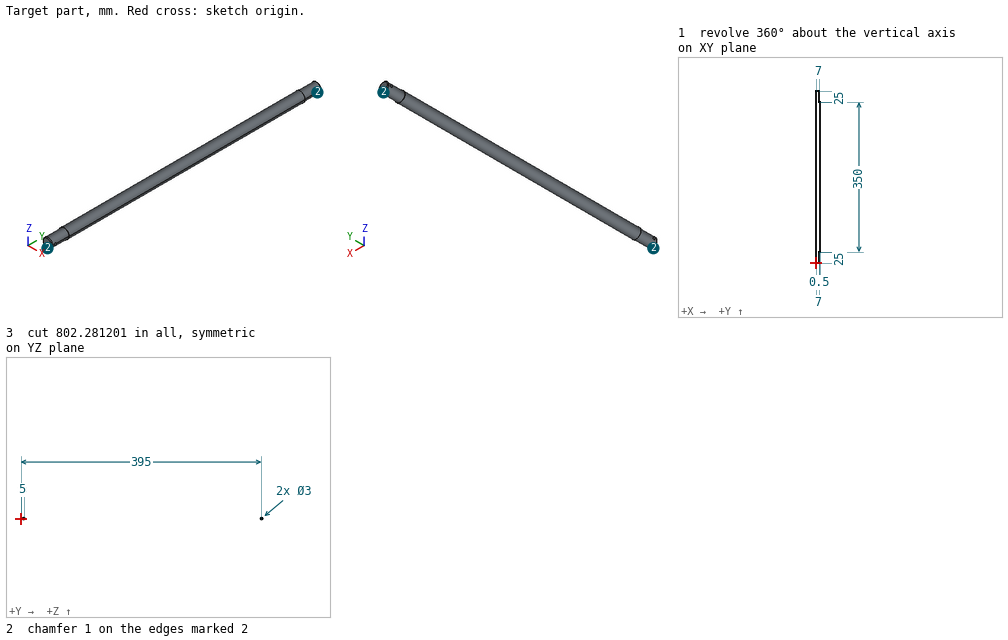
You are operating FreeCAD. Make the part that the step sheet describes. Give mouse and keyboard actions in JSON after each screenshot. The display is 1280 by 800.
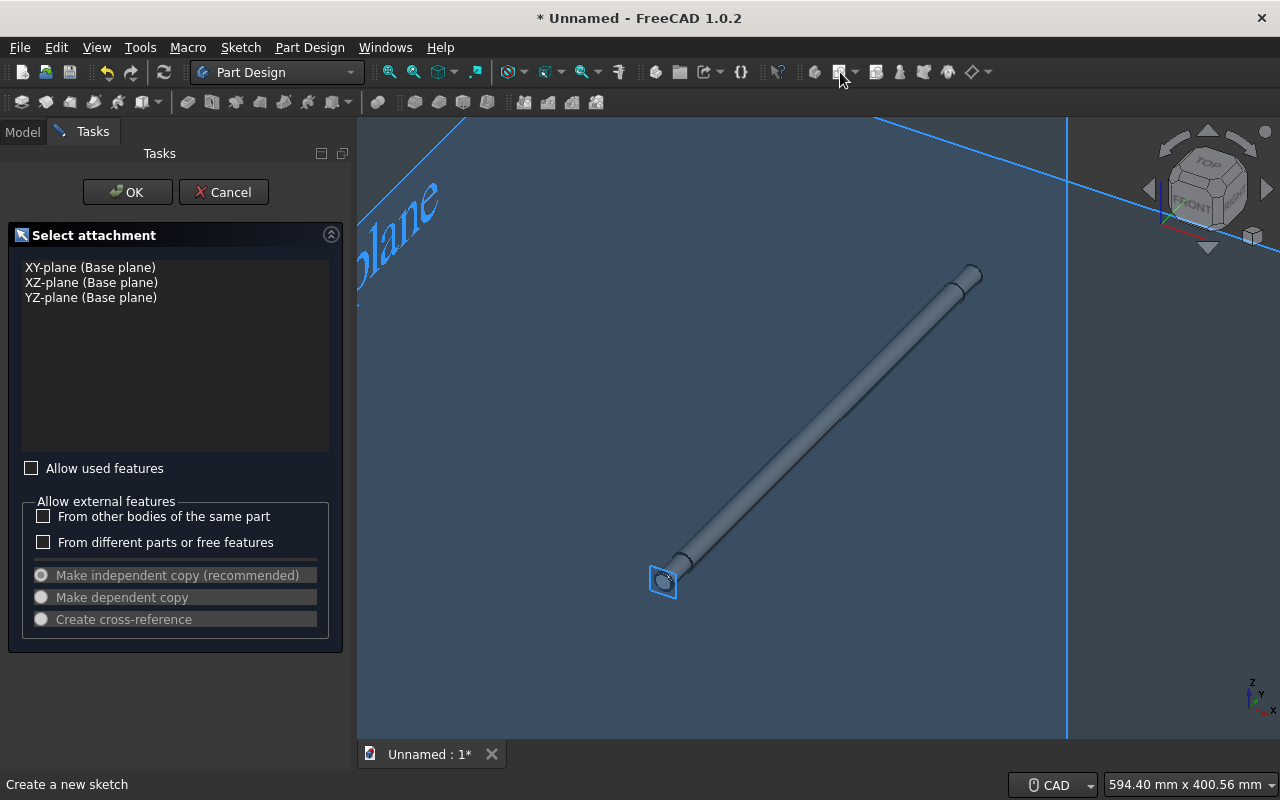
{"action": "left_click", "coordinate": [82, 298]}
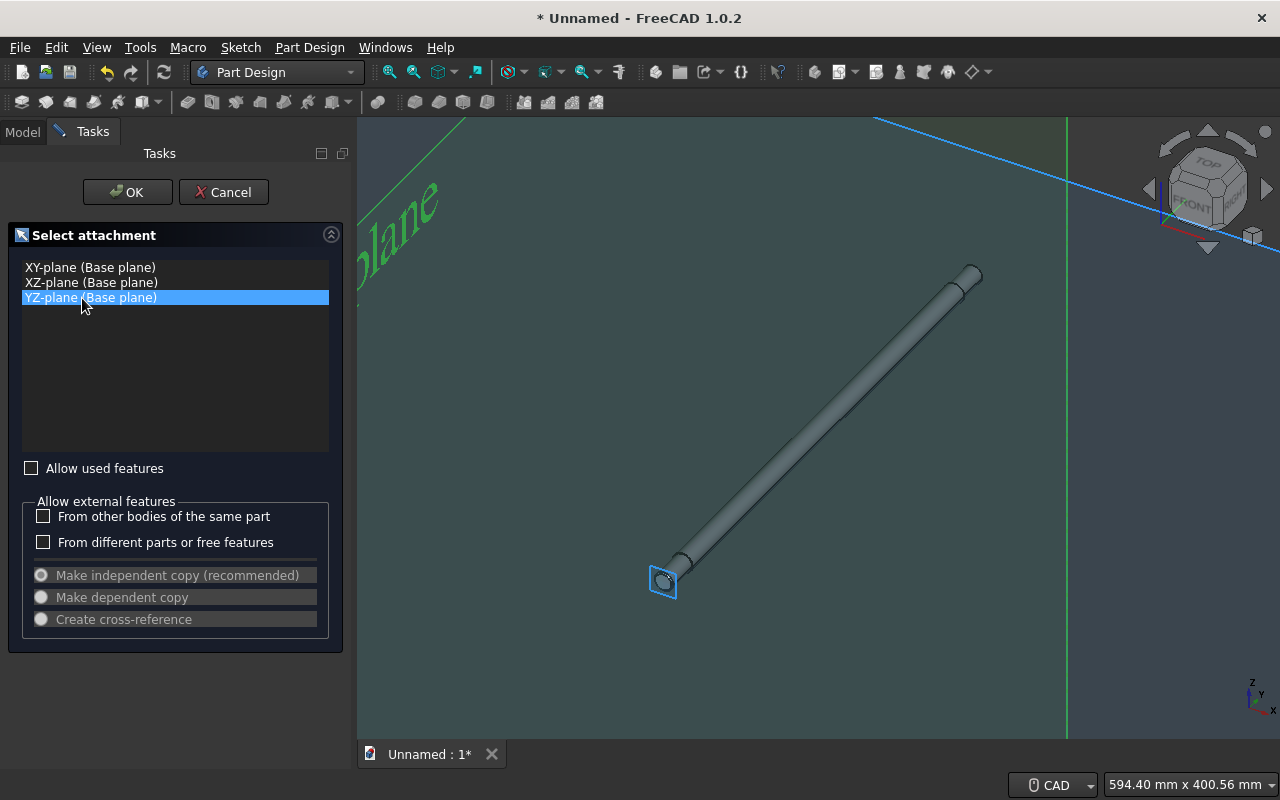
{"action": "left_click", "coordinate": [128, 192]}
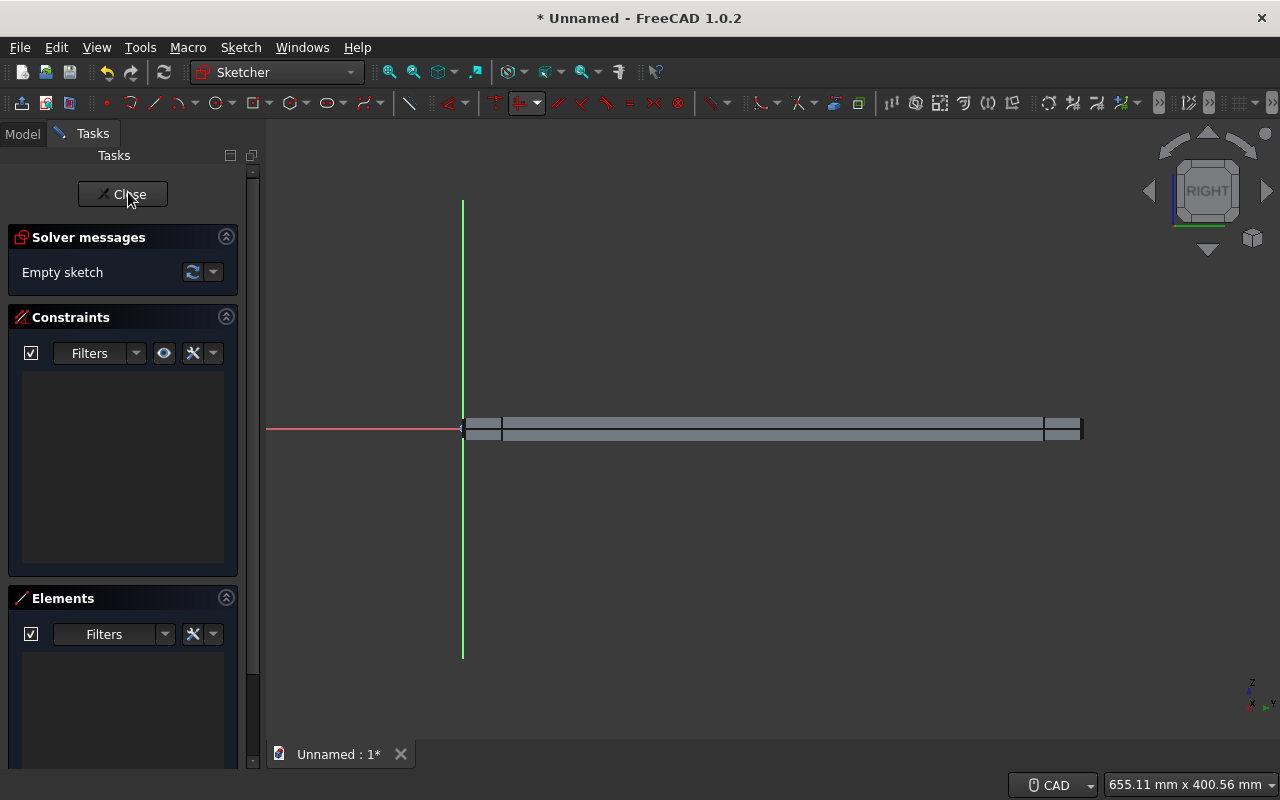
{"action": "left_click", "coordinate": [70, 104]}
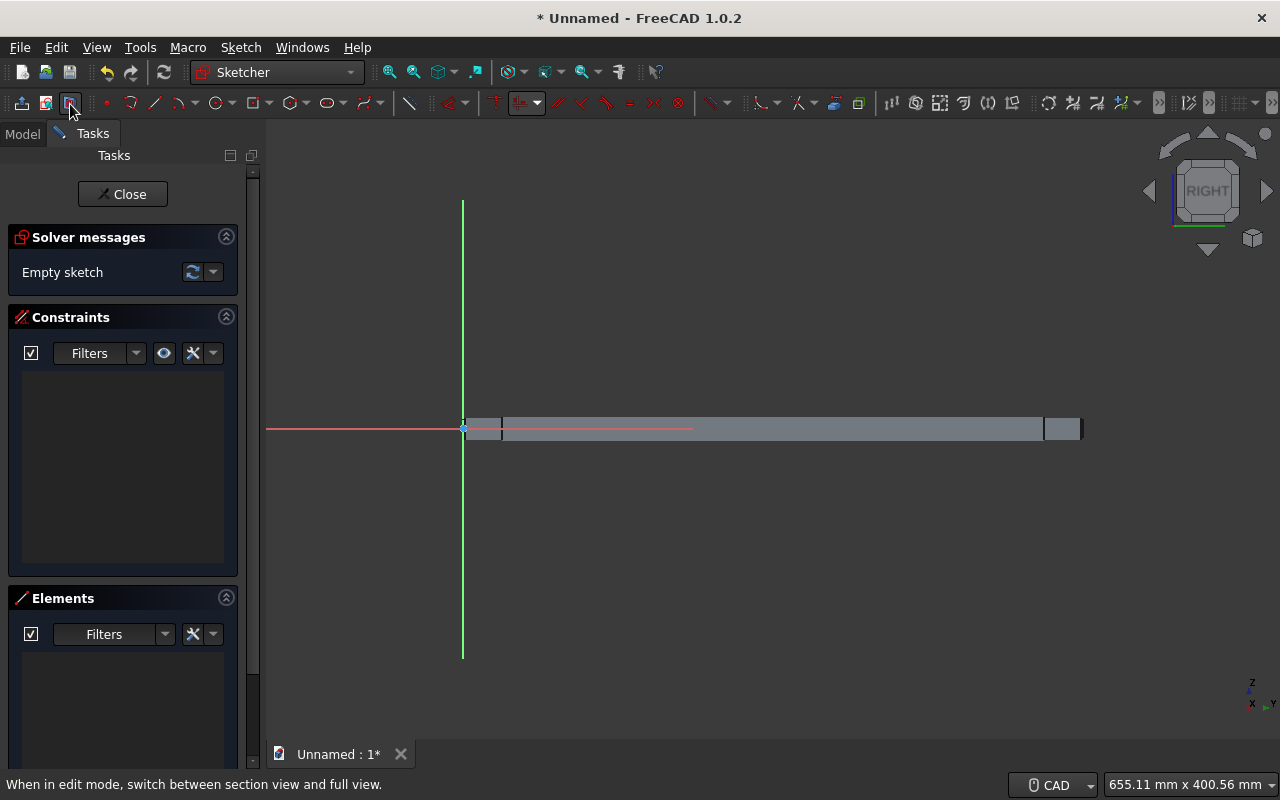
{"action": "key", "text": "g c"}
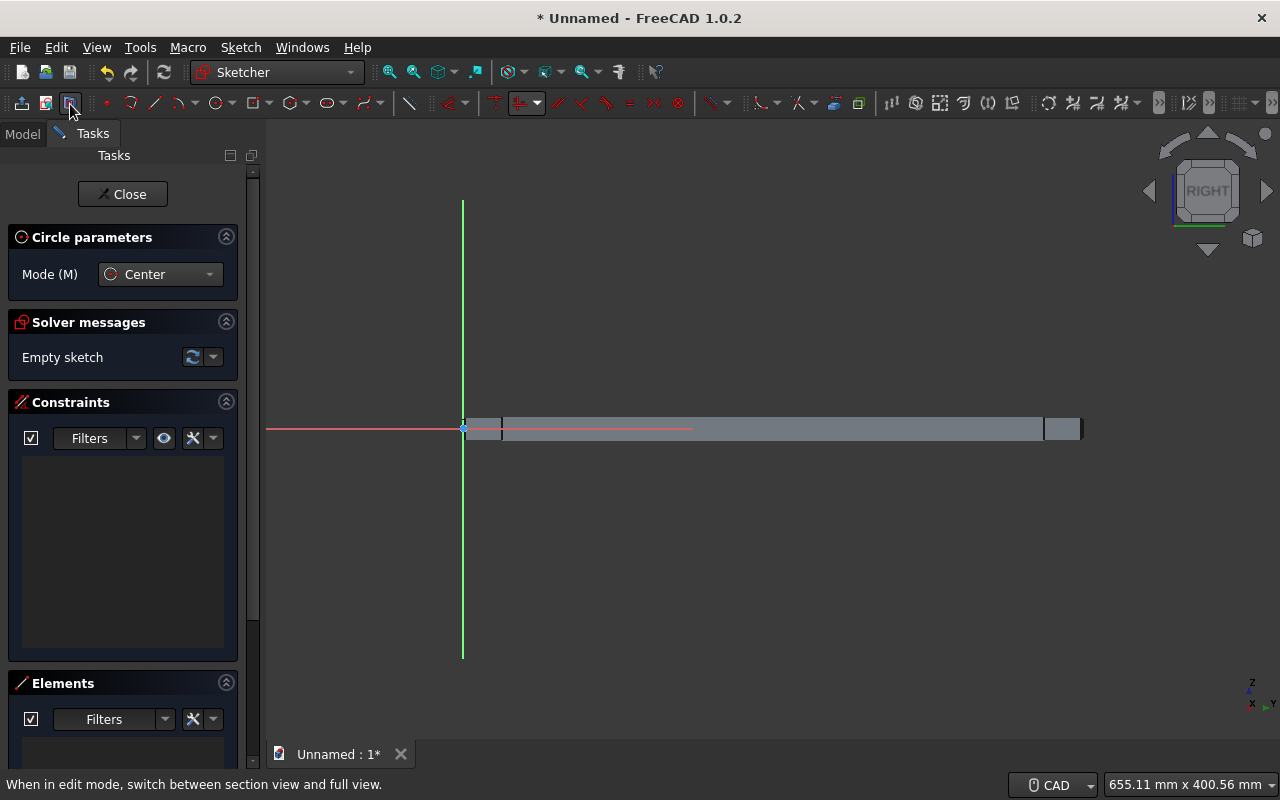
{"action": "scroll", "coordinate": [1075, 429], "scroll_direction": "up", "scroll_amount": 12}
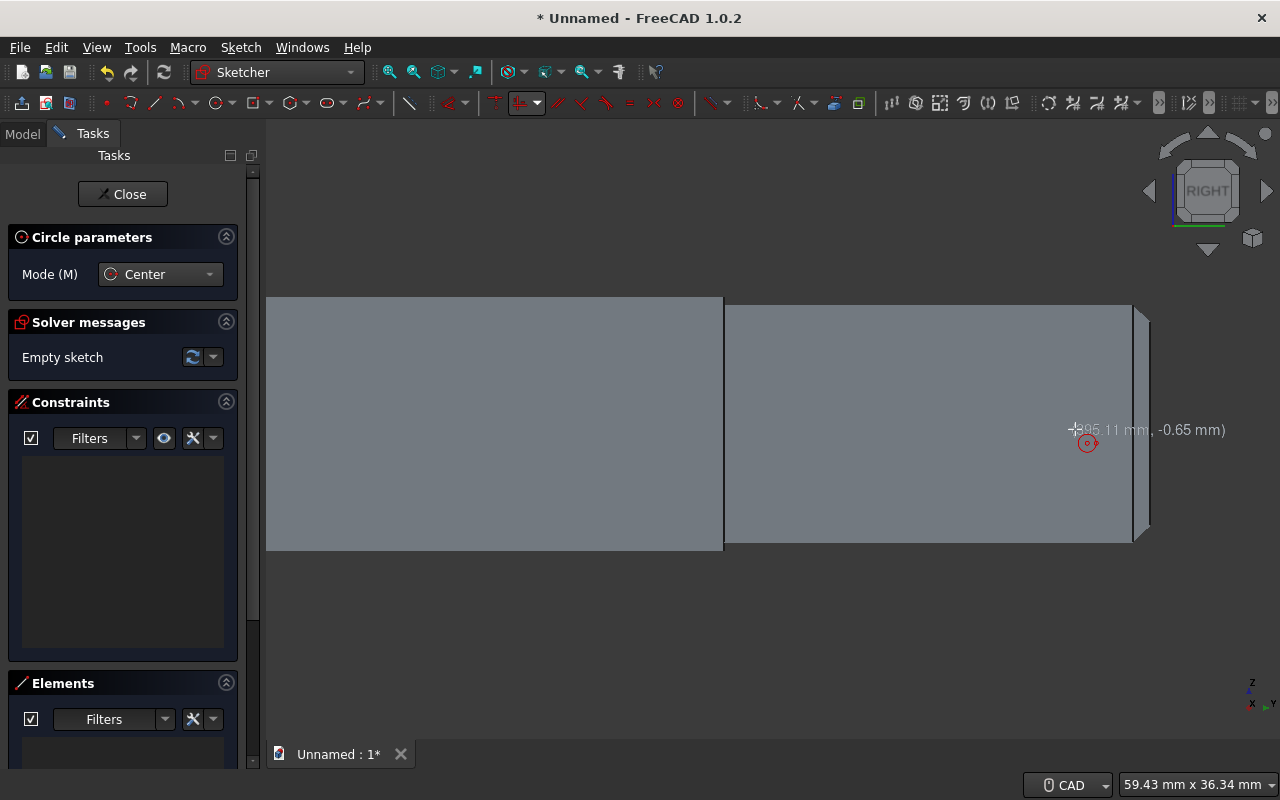
{"action": "scroll", "coordinate": [1003, 430], "scroll_direction": "down", "scroll_amount": 12}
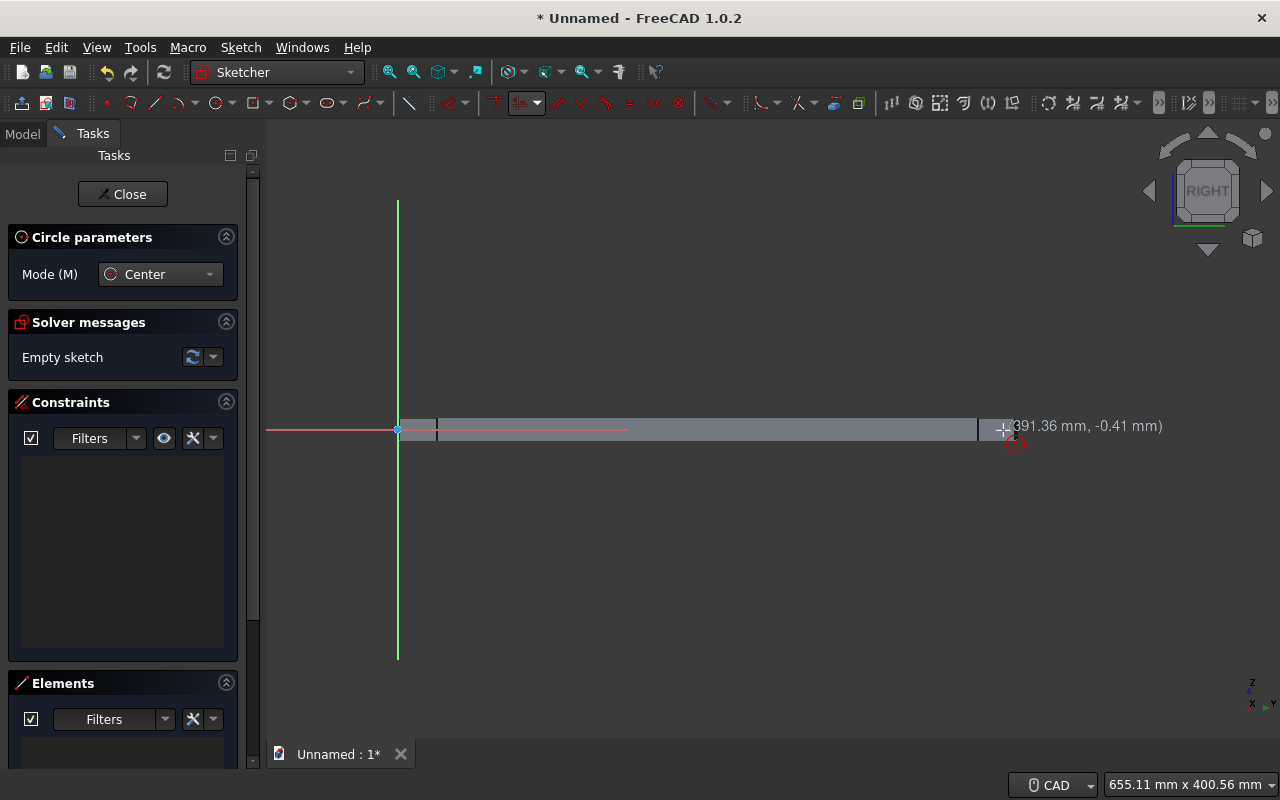
{"action": "left_click", "coordinate": [1009, 430]}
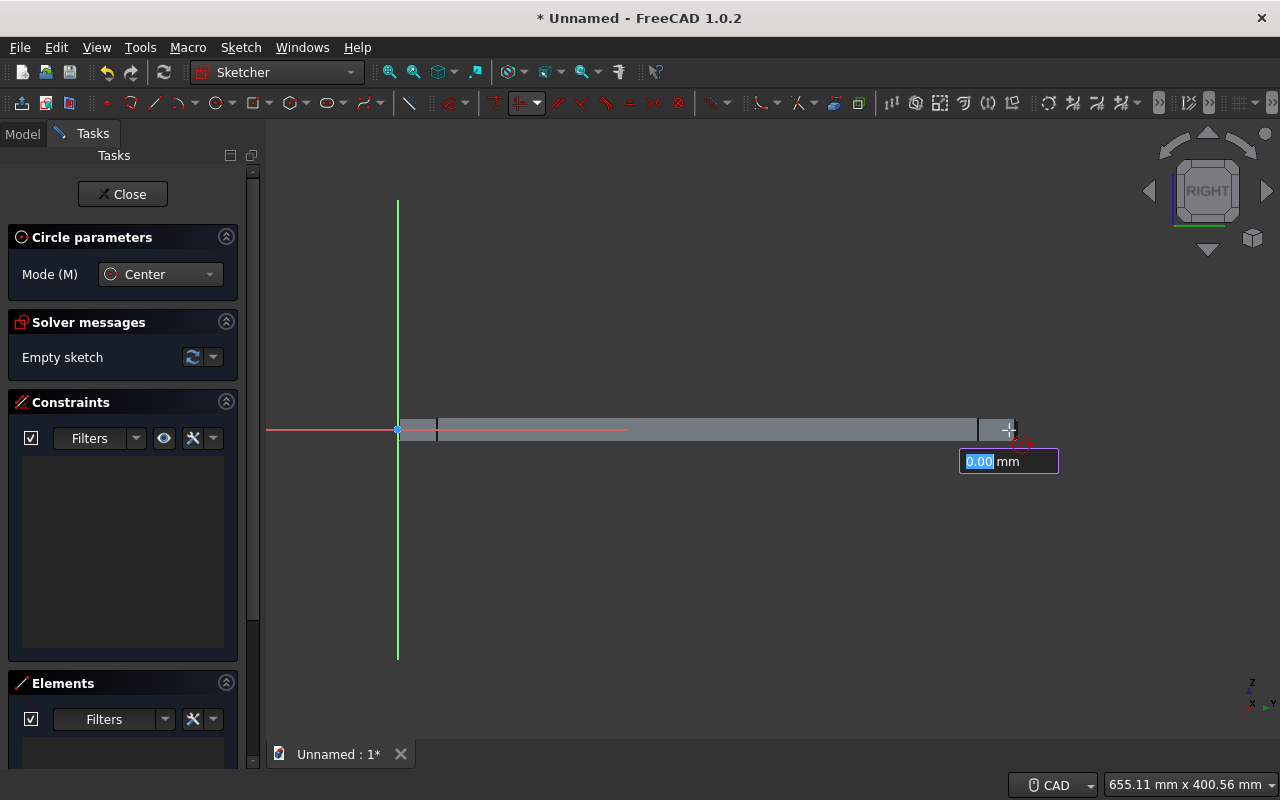
{"action": "scroll", "coordinate": [1009, 432], "scroll_direction": "up", "scroll_amount": 10}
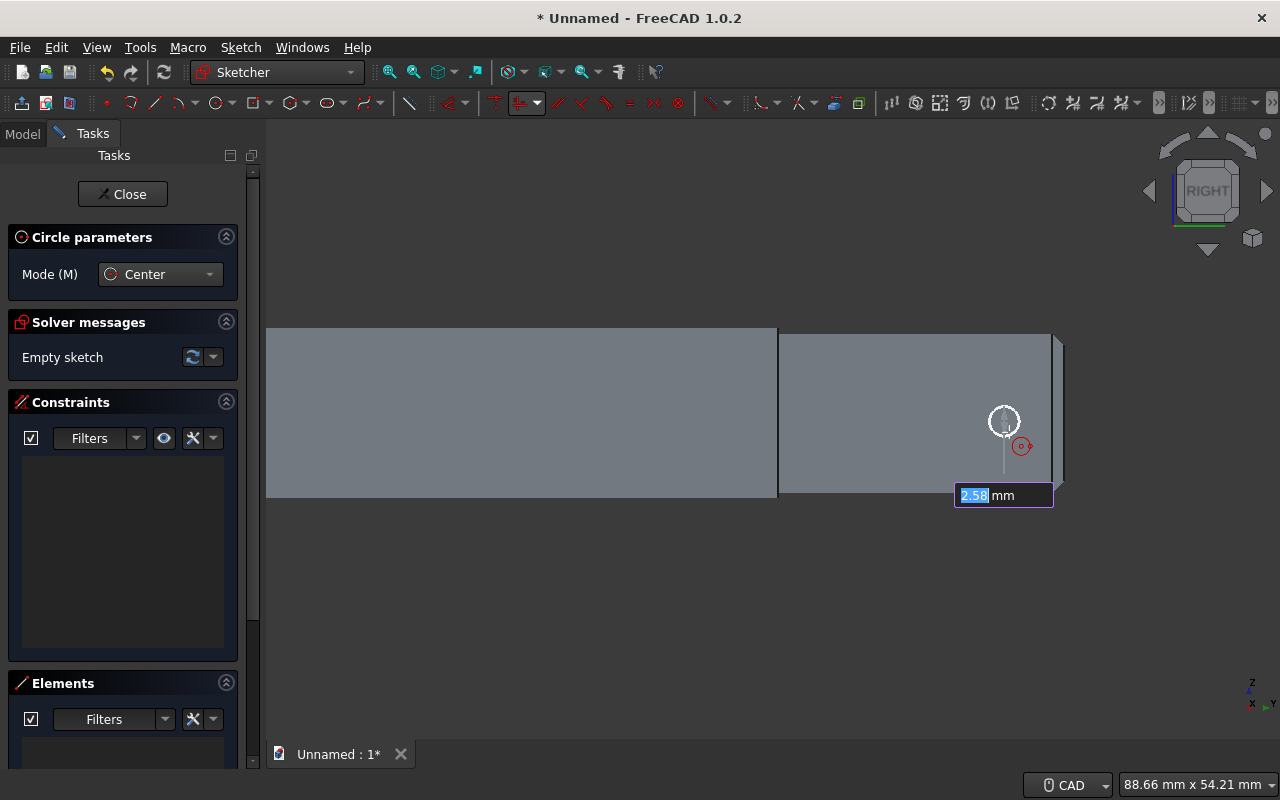
{"action": "left_click", "coordinate": [1001, 429]}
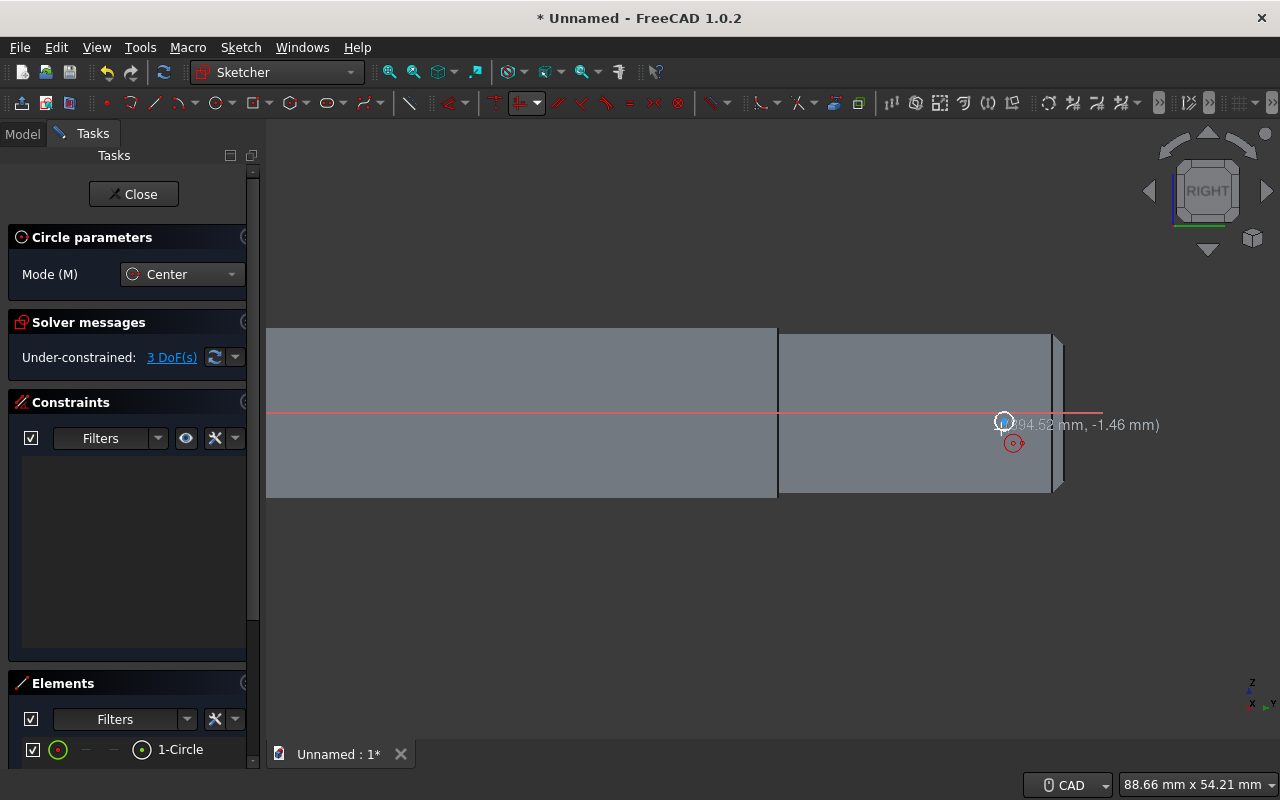
{"action": "scroll", "coordinate": [1009, 431], "scroll_direction": "down", "scroll_amount": 10}